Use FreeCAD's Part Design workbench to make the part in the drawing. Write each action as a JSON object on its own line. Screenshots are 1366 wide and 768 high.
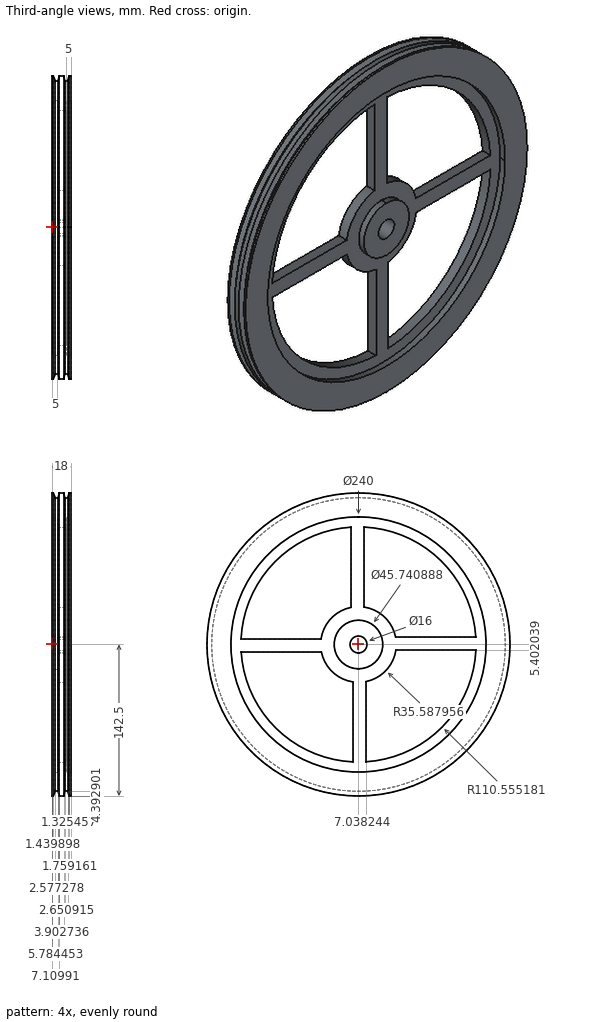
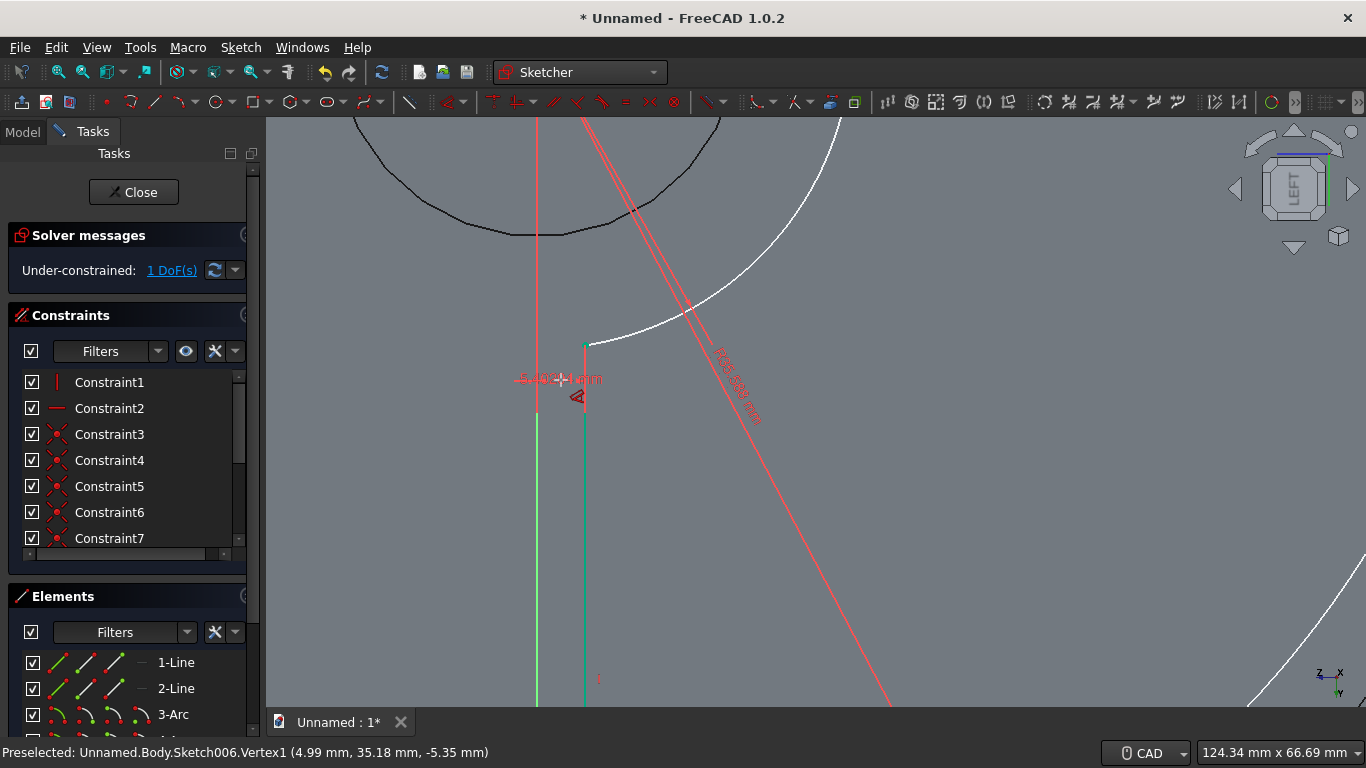
{"action": "scroll", "coordinate": [586, 348], "scroll_direction": "down", "scroll_amount": 5}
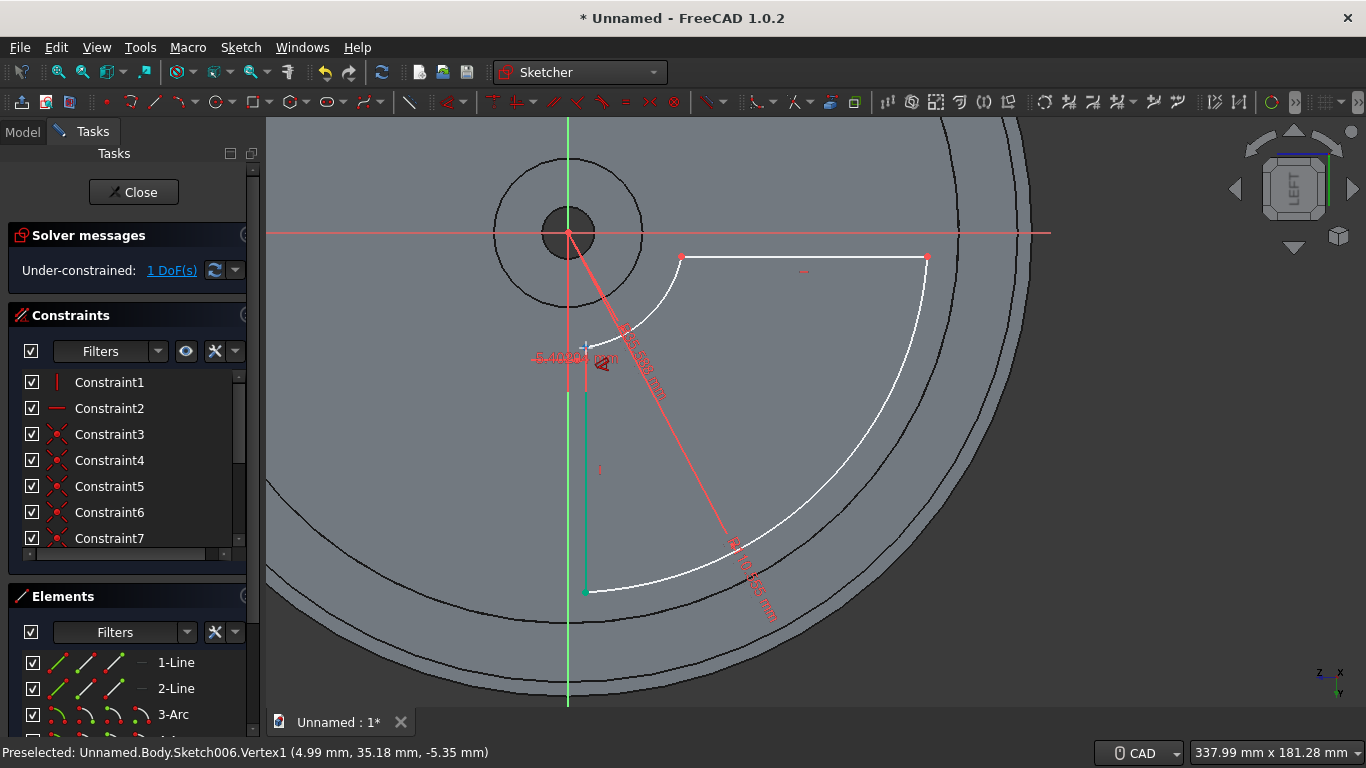
{"action": "scroll", "coordinate": [927, 257], "scroll_direction": "up", "scroll_amount": 3}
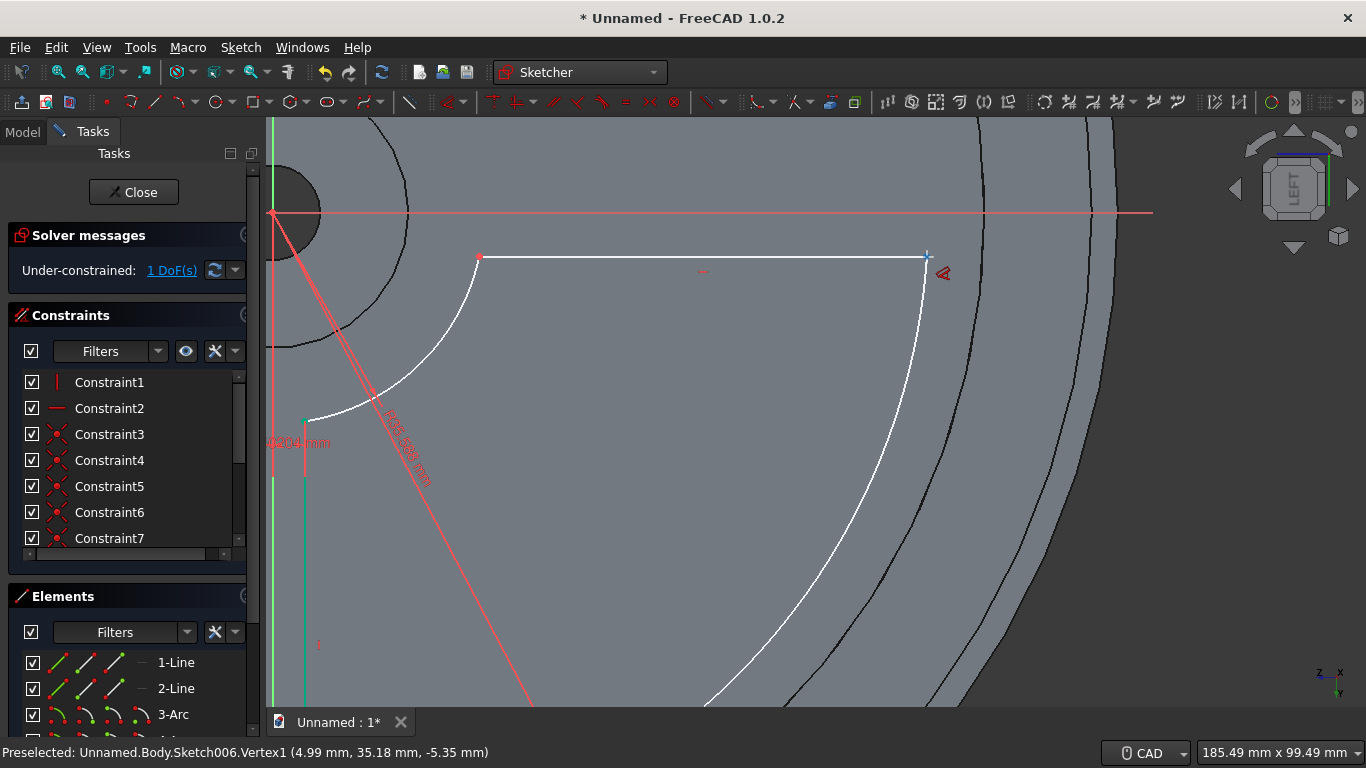
{"action": "left_click", "coordinate": [927, 257]}
{"action": "left_click", "coordinate": [961, 235]}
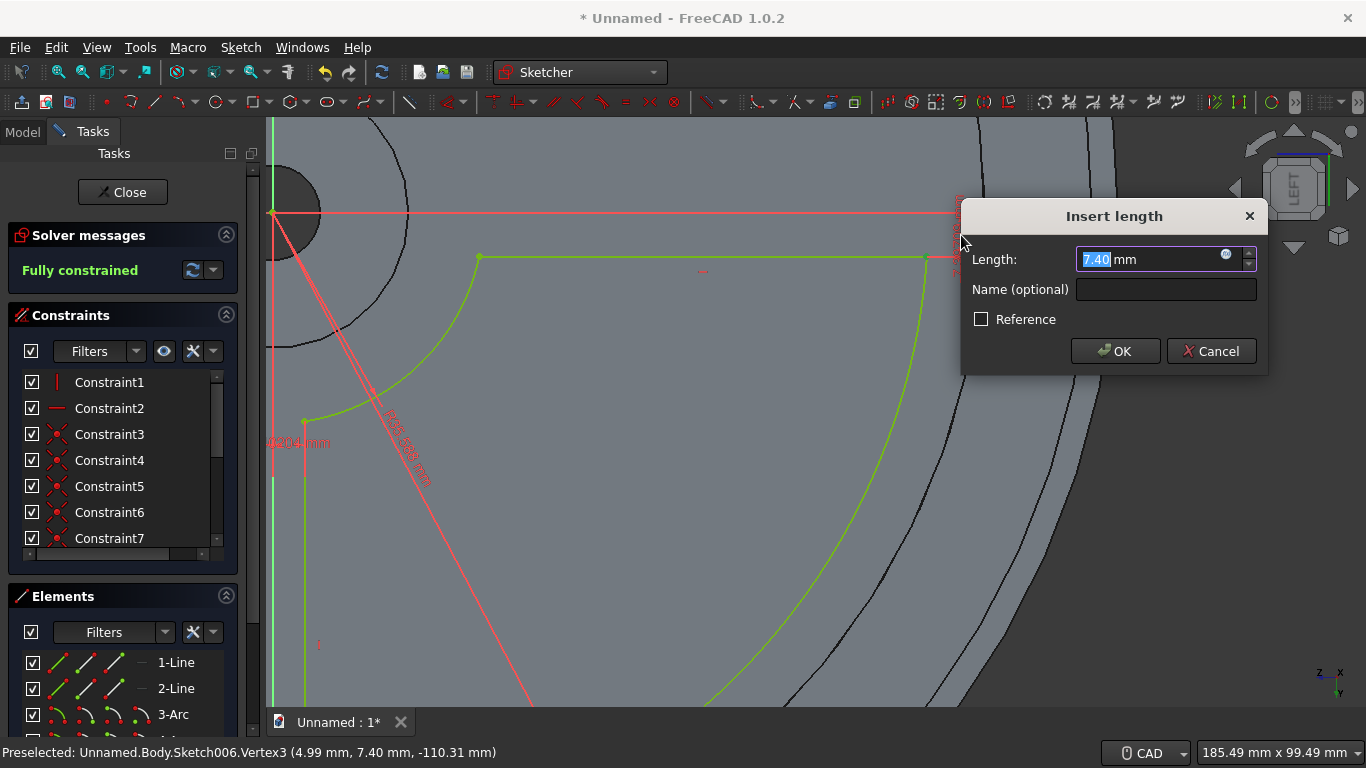
{"action": "type", "text": "7.038244"}
{"action": "key", "text": "Return"}
{"action": "key", "text": "Escape"}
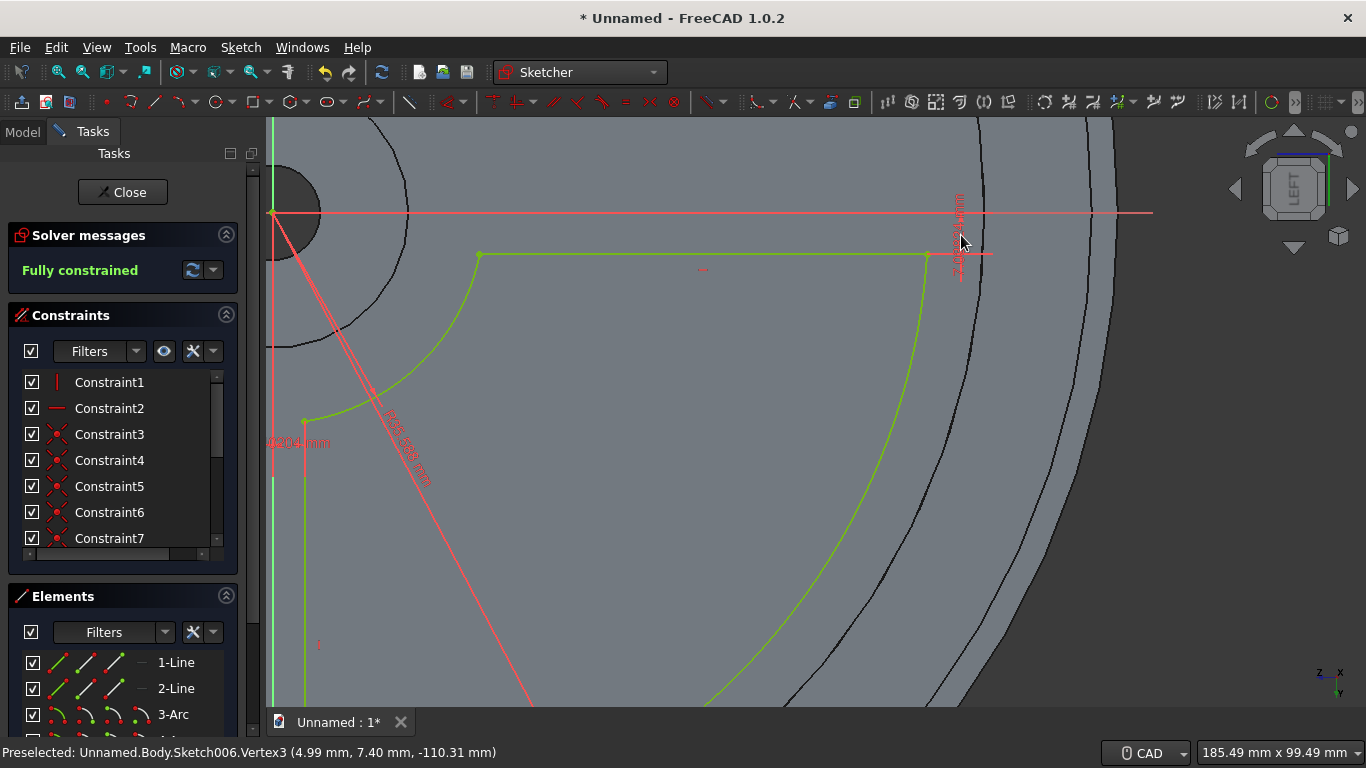
{"action": "left_click", "coordinate": [123, 192]}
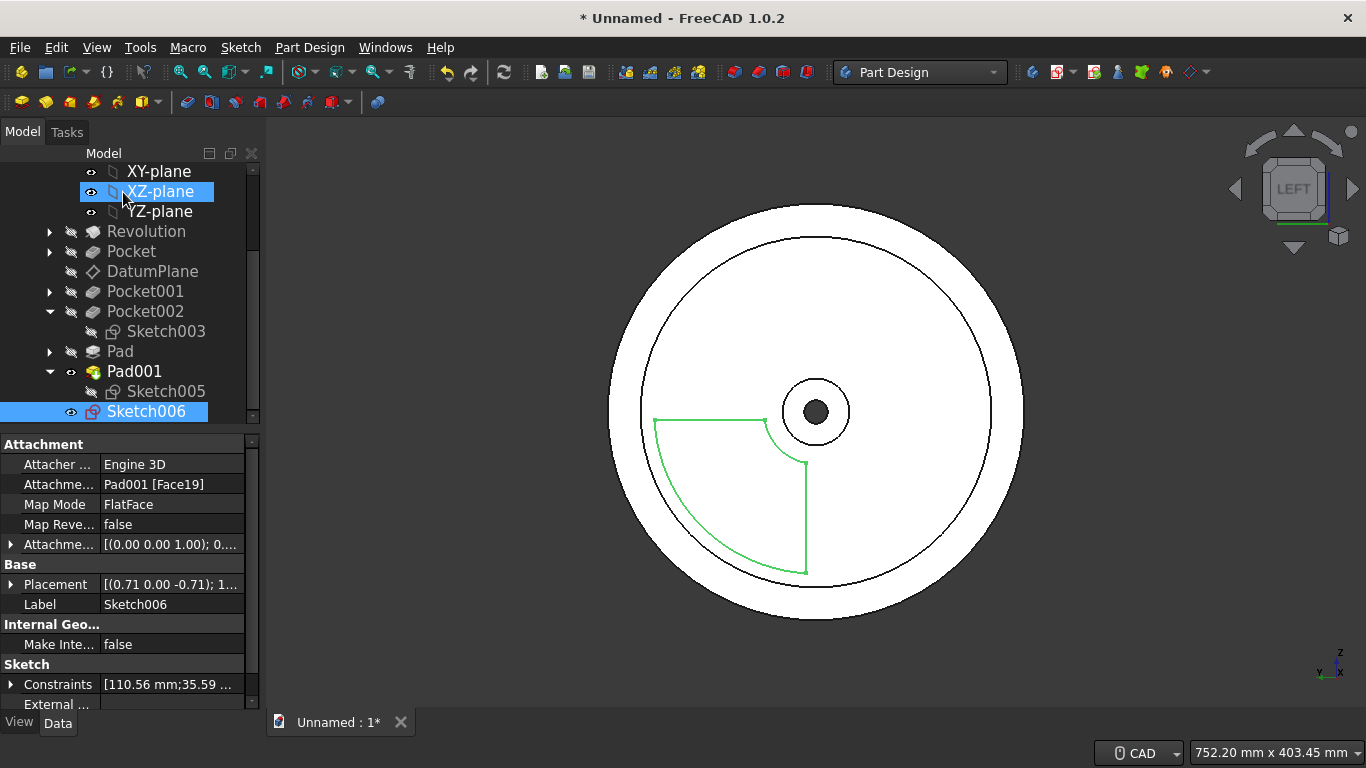
{"action": "left_click", "coordinate": [188, 102]}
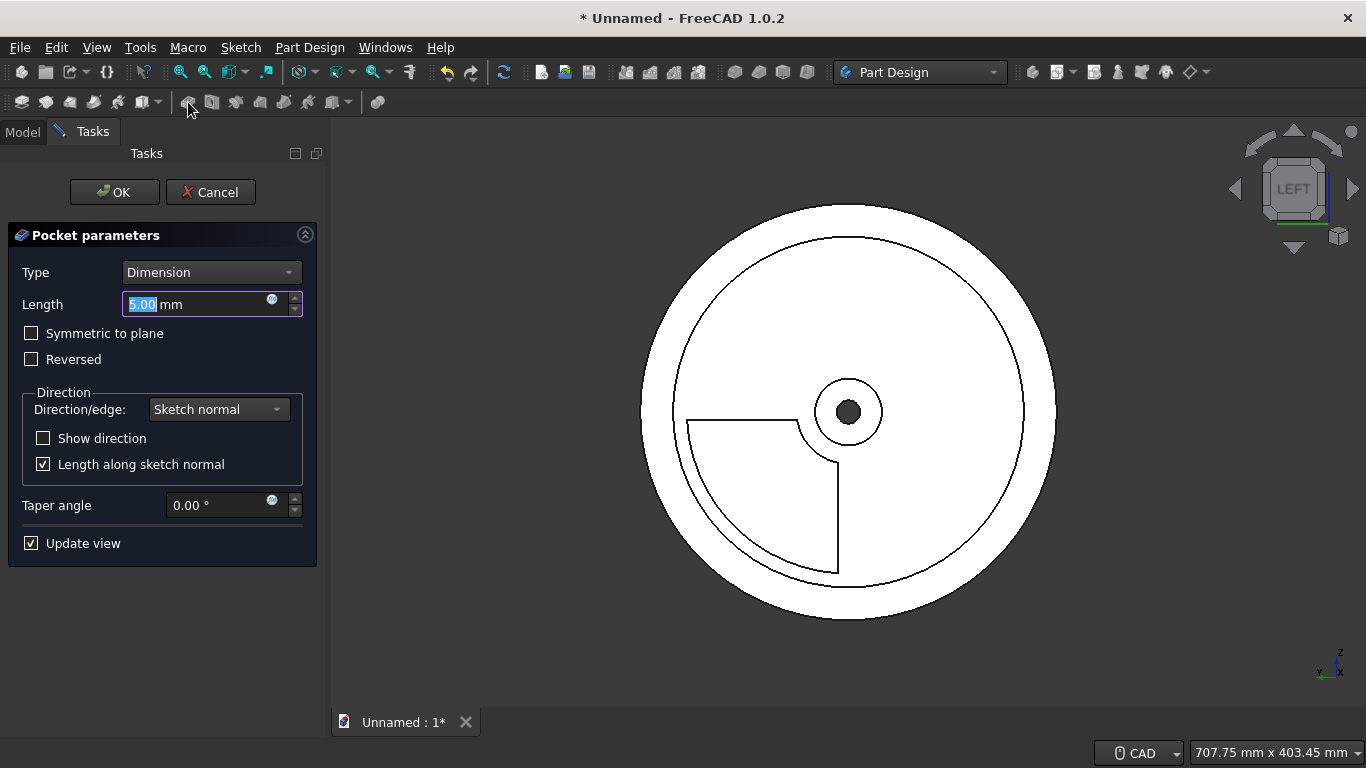
{"action": "left_click", "coordinate": [212, 272]}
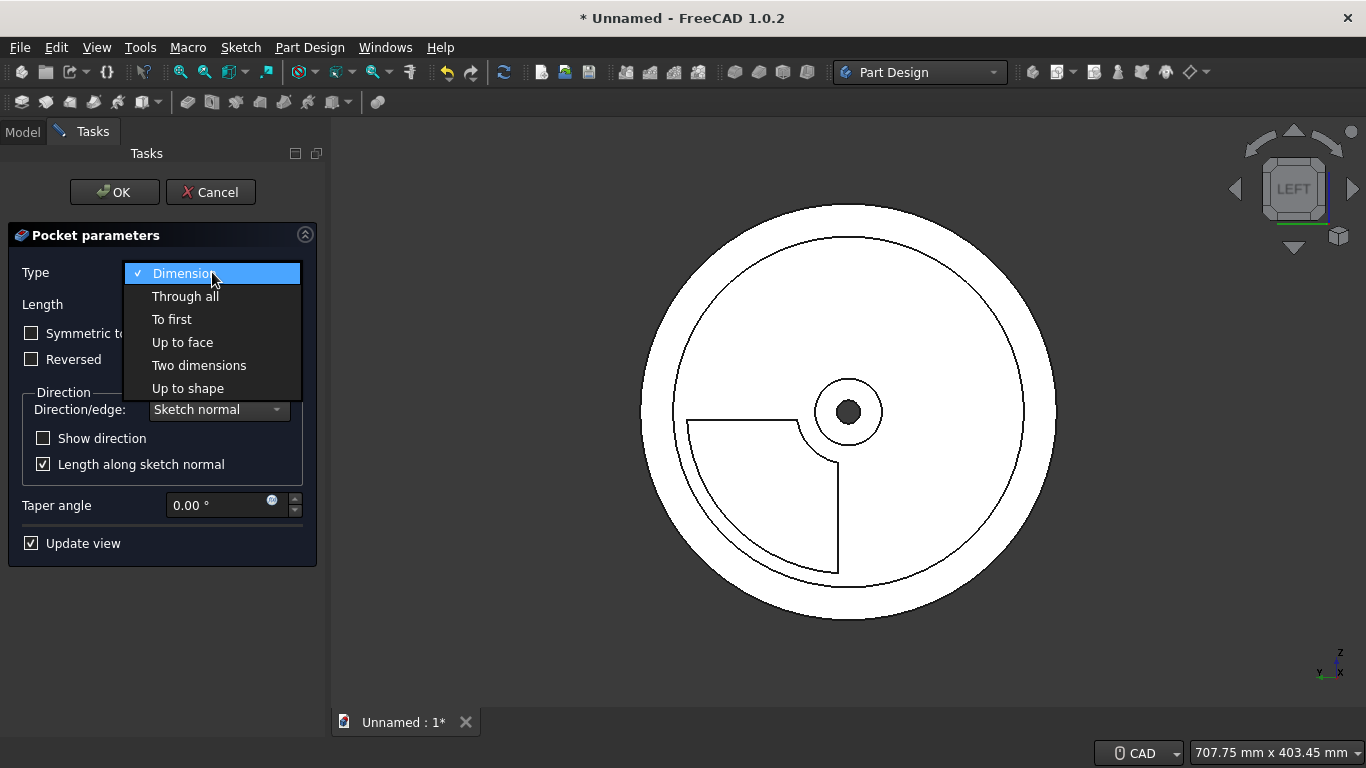
{"action": "left_click", "coordinate": [212, 296]}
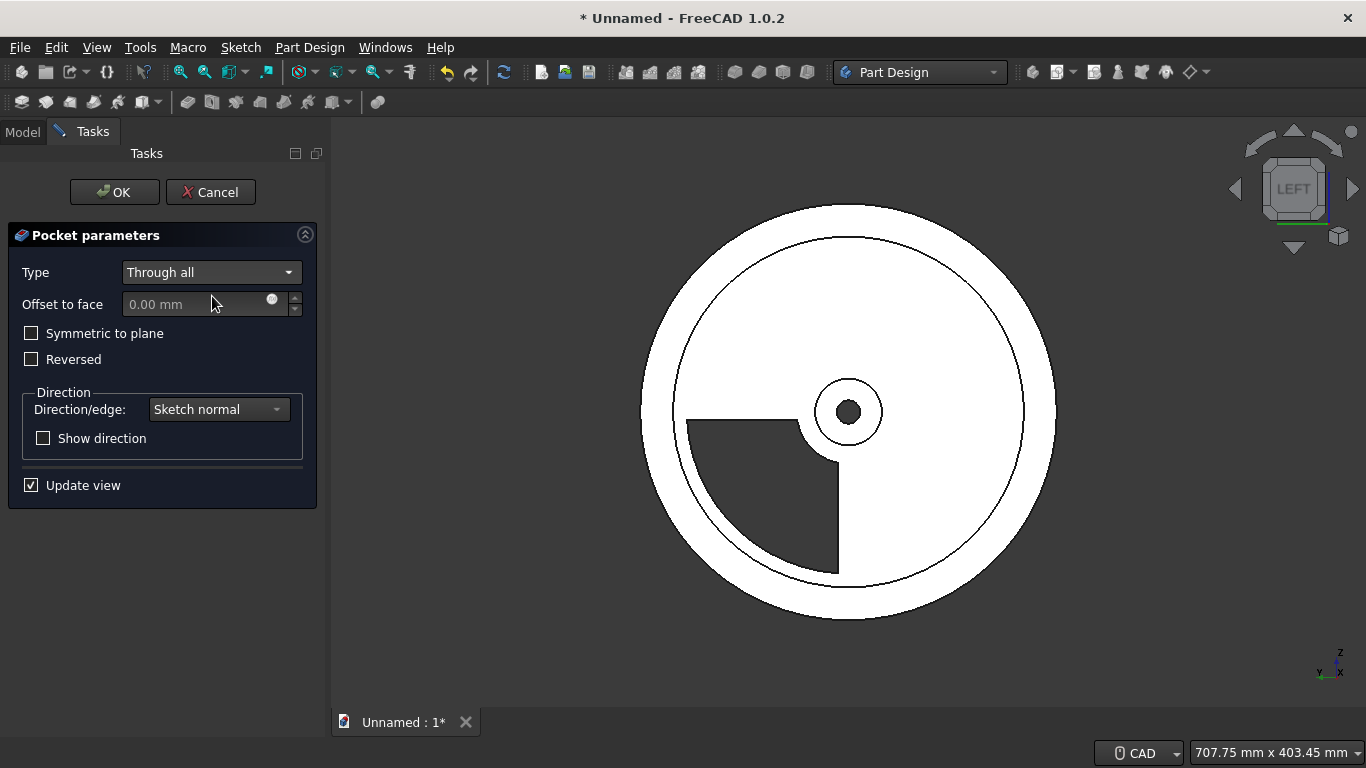
{"action": "left_click", "coordinate": [115, 192]}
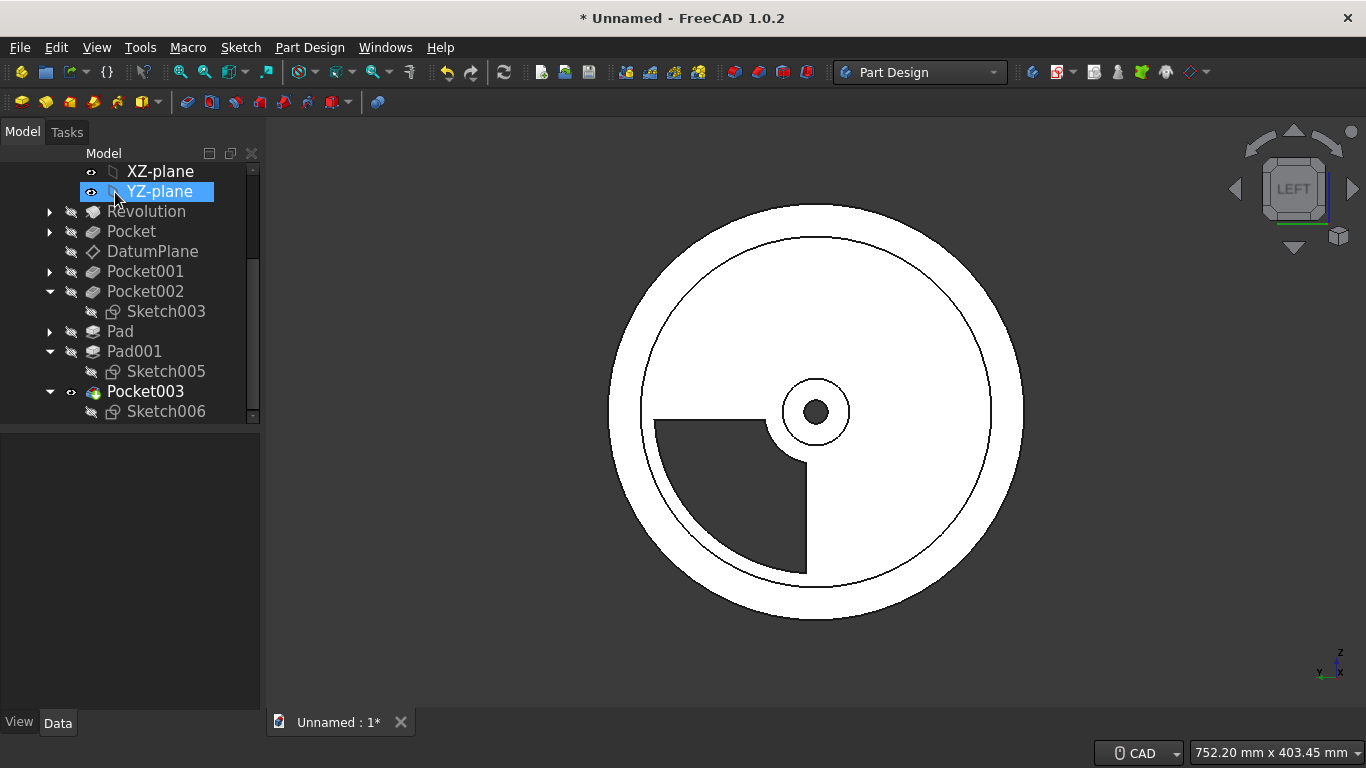
{"action": "left_click", "coordinate": [116, 392]}